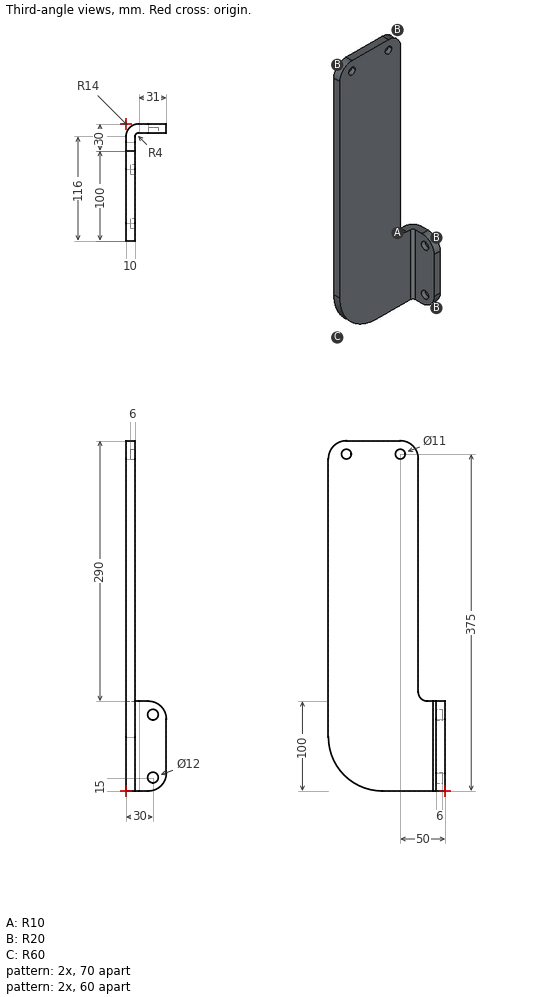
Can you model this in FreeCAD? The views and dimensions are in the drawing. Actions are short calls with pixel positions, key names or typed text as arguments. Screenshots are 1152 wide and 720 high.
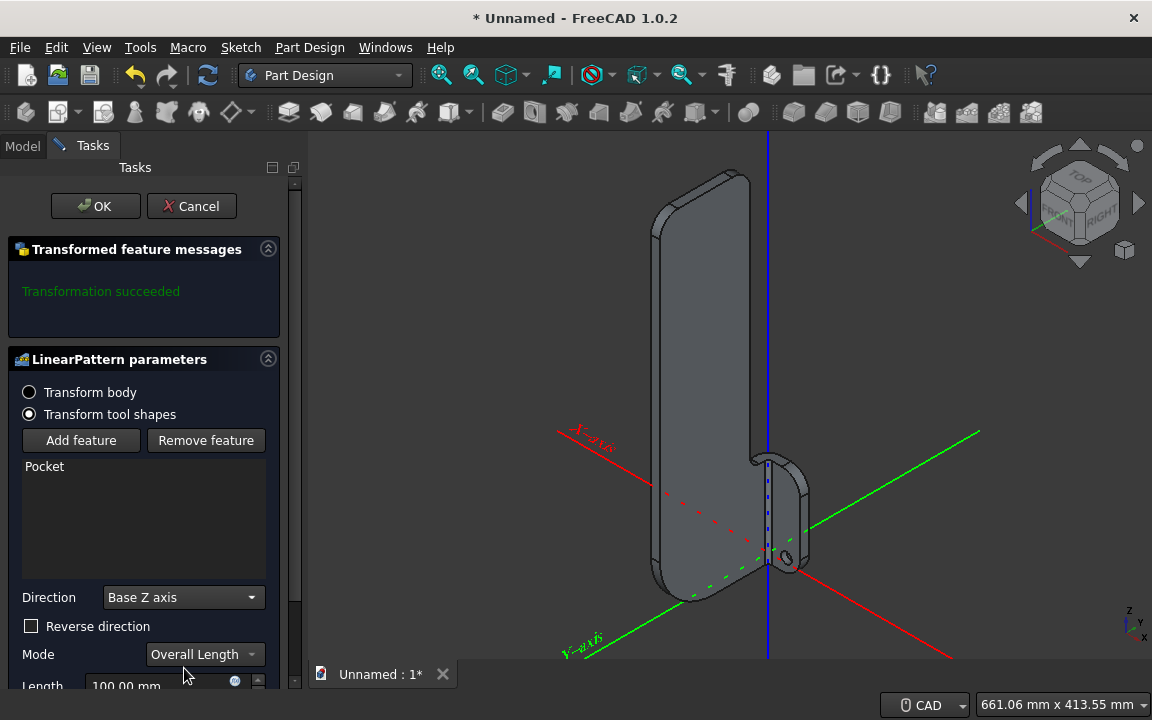
click(206, 654)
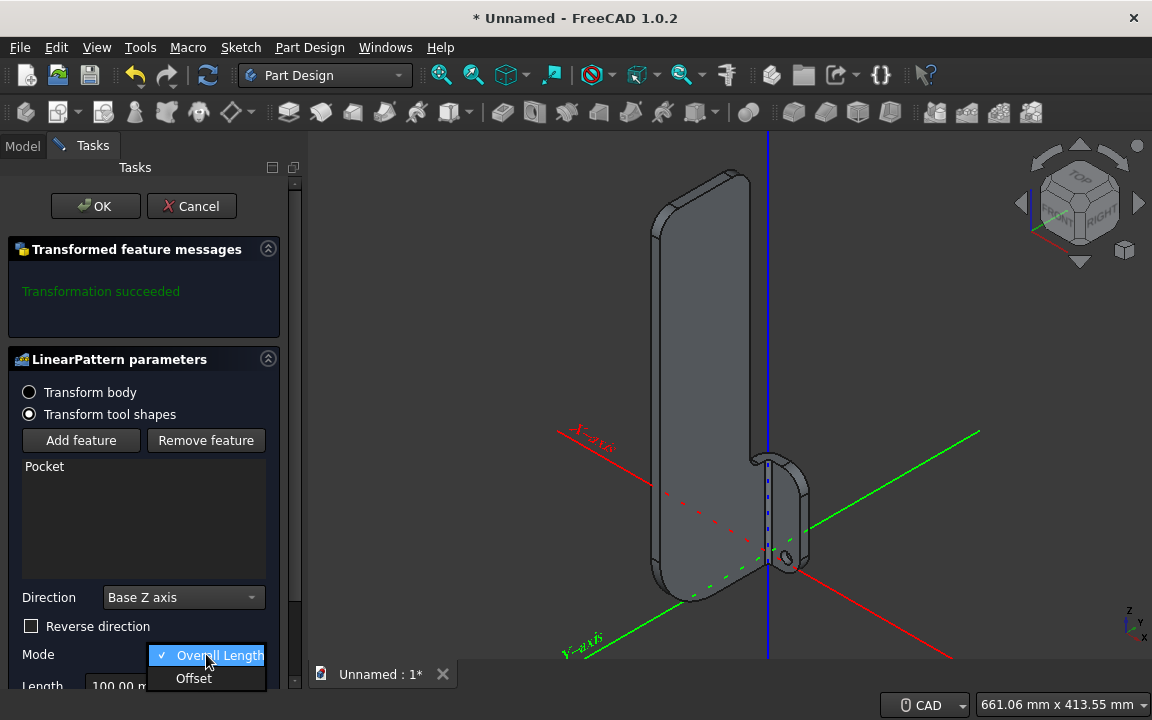
click(206, 678)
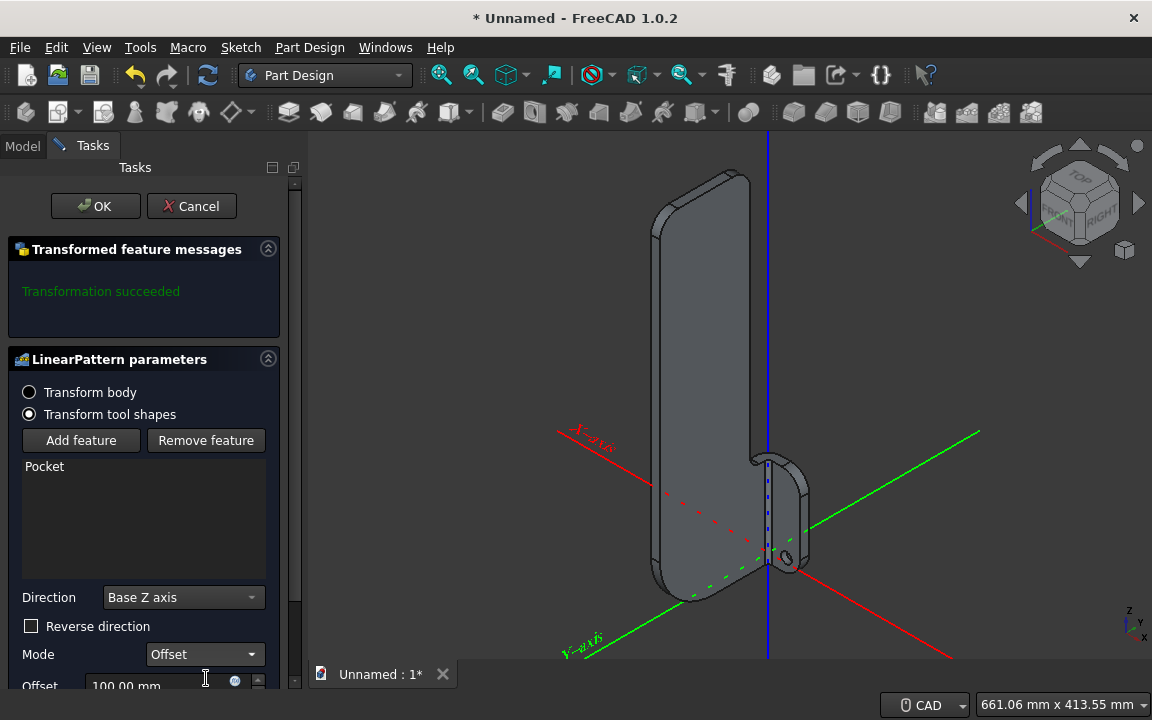
scroll(295, 432, down, 2)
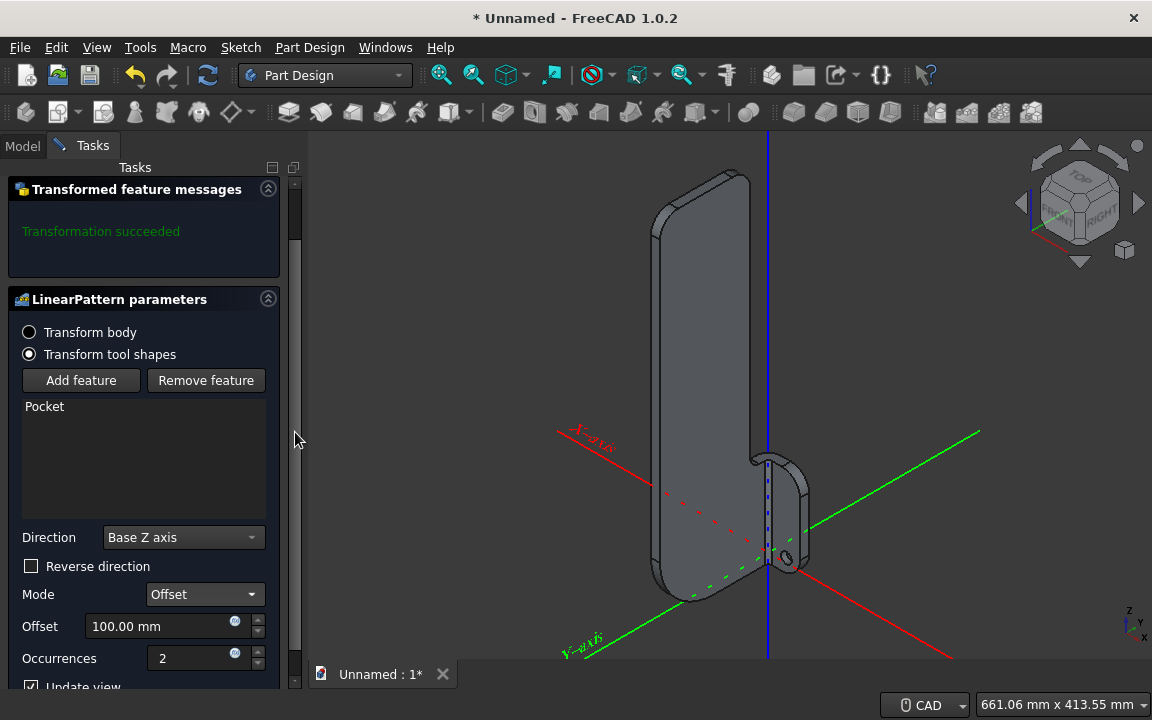
triple_click(168, 596)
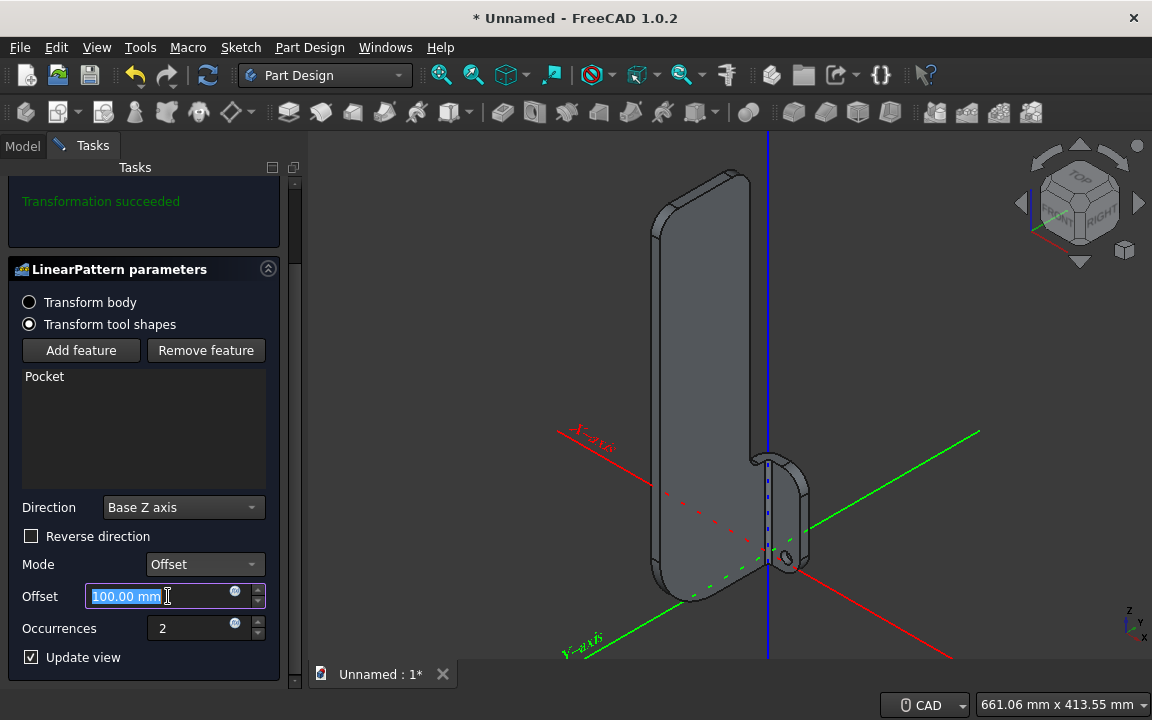
text(70)
key(Tab)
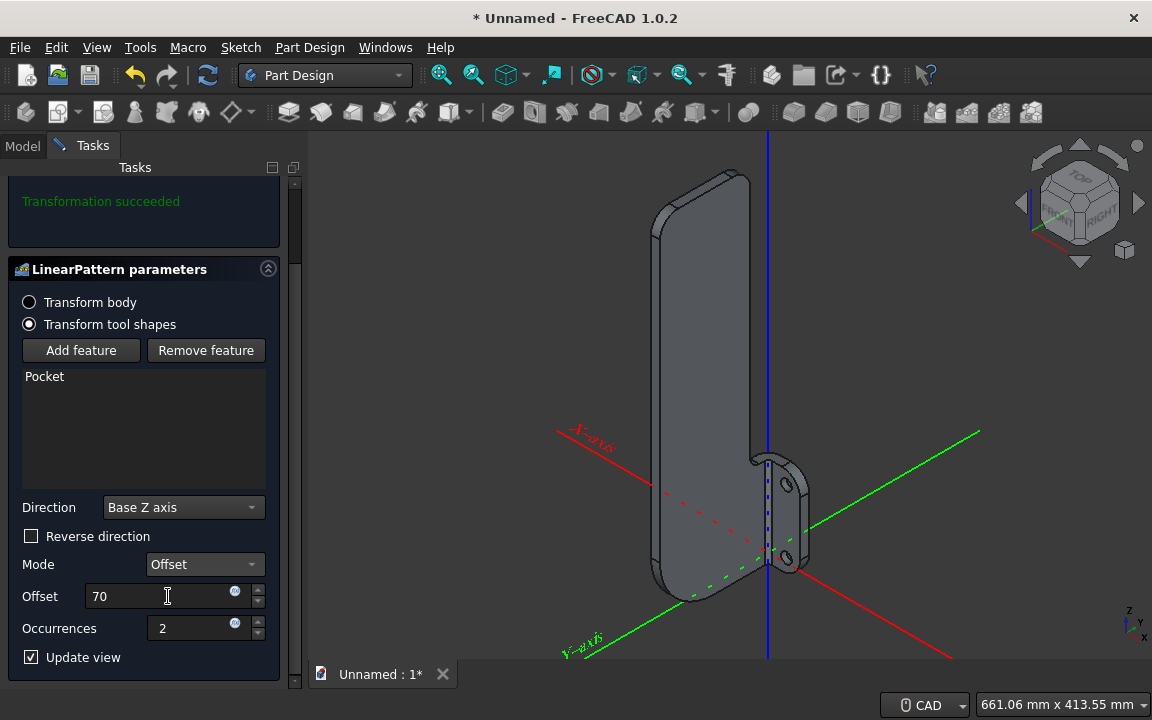
triple_click(198, 628)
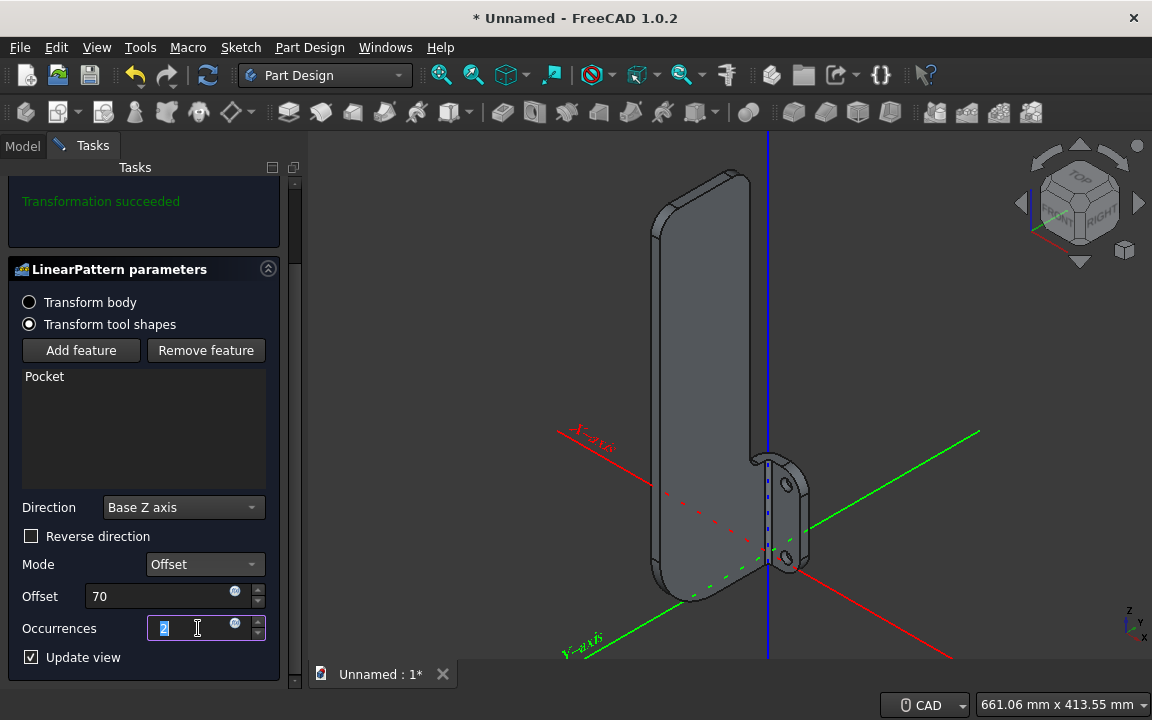
text(2)
key(Tab)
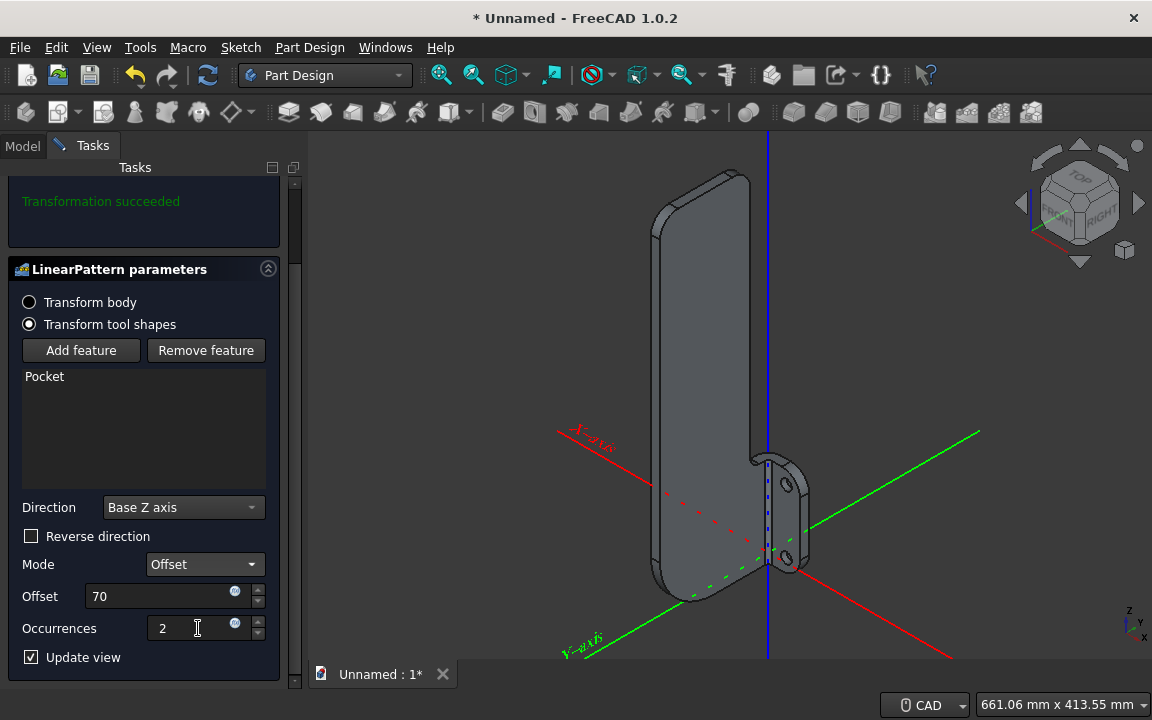
scroll(295, 432, up, 3)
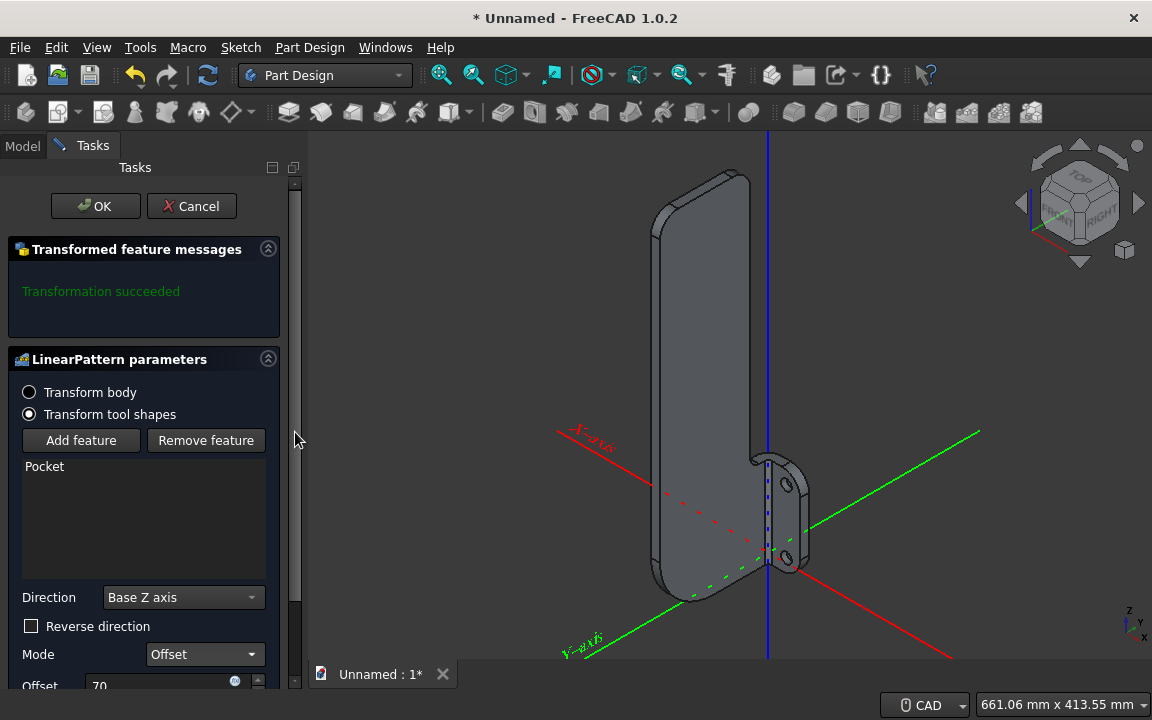
click(96, 206)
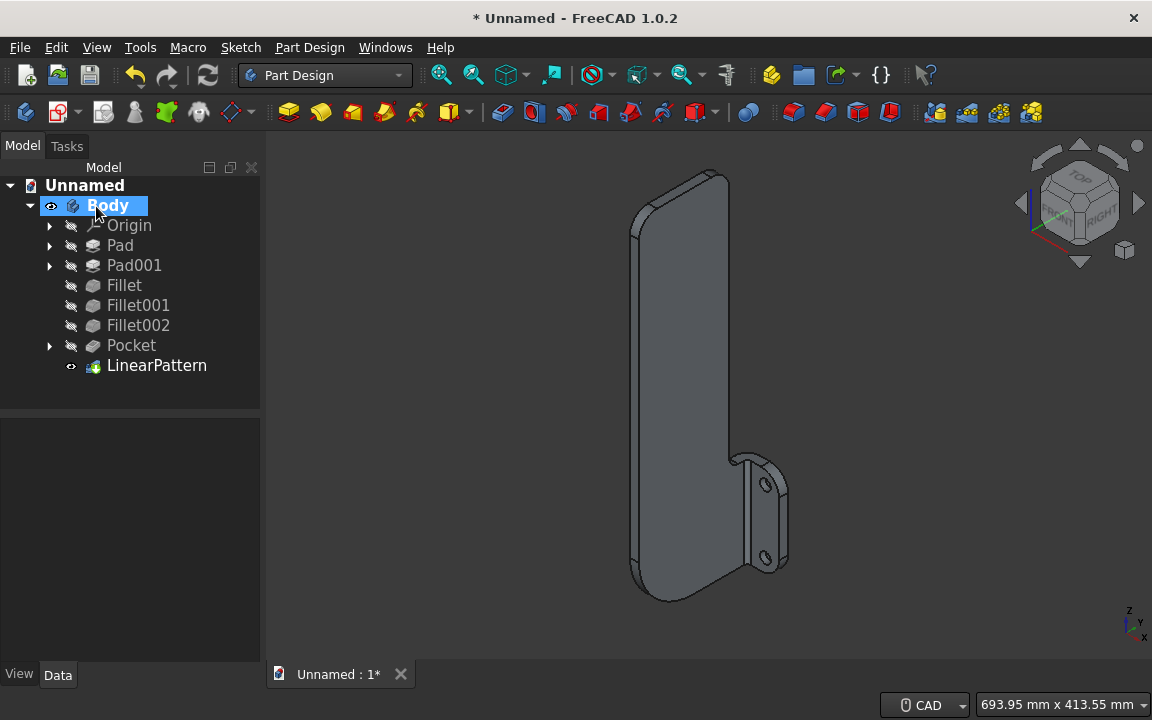
click(691, 507)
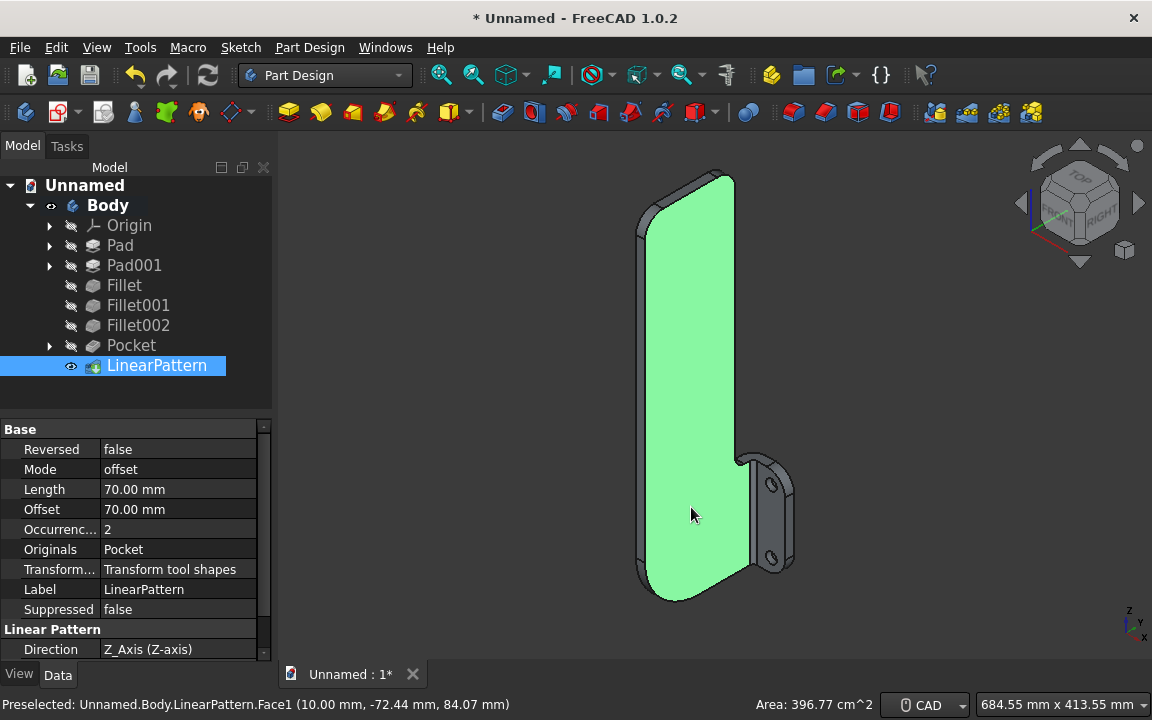
click(58, 112)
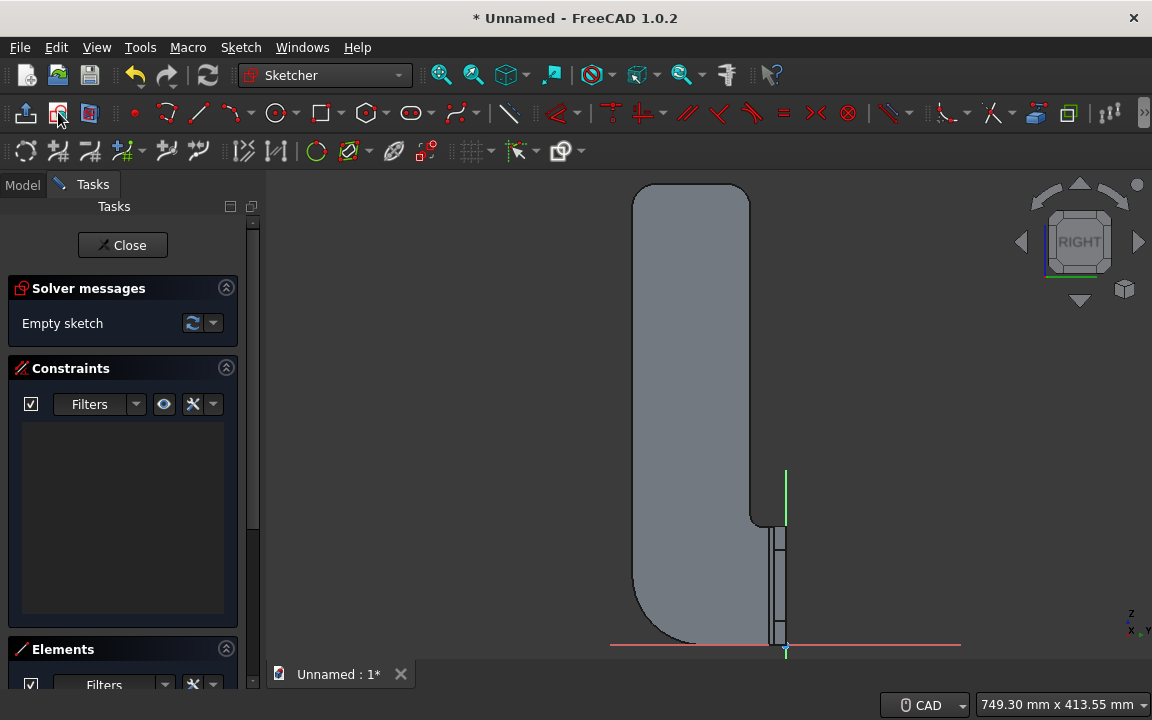
scroll(640, 414, down, 5)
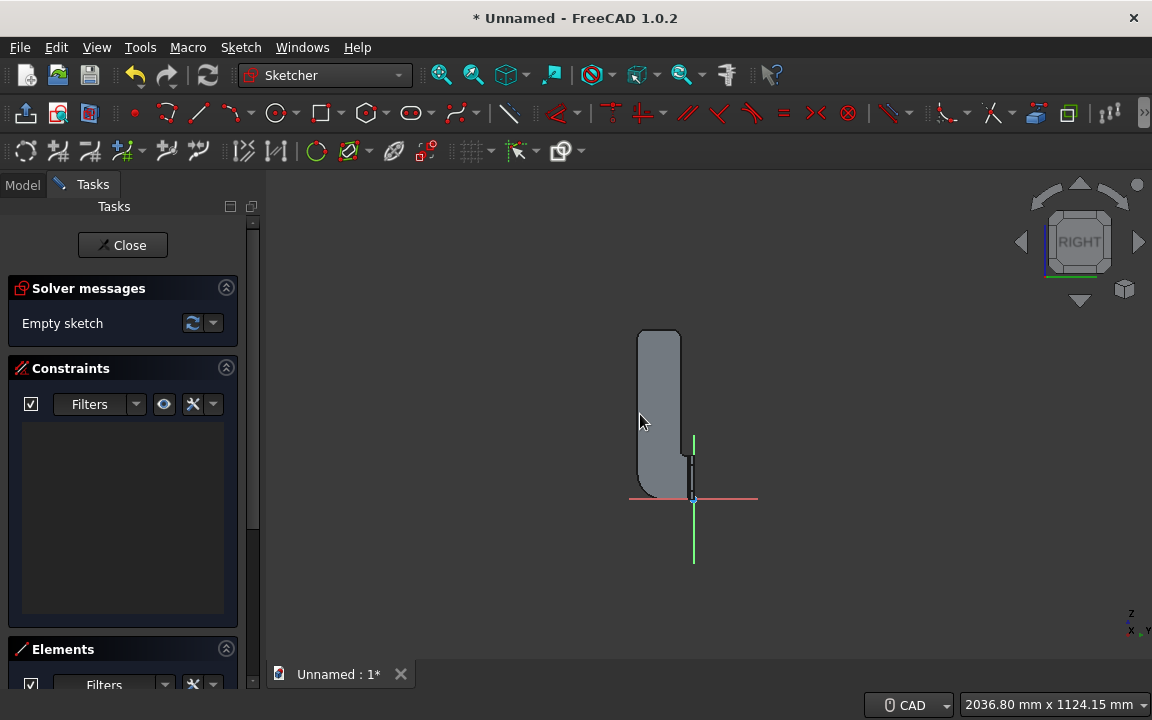
scroll(674, 332, up, 15)